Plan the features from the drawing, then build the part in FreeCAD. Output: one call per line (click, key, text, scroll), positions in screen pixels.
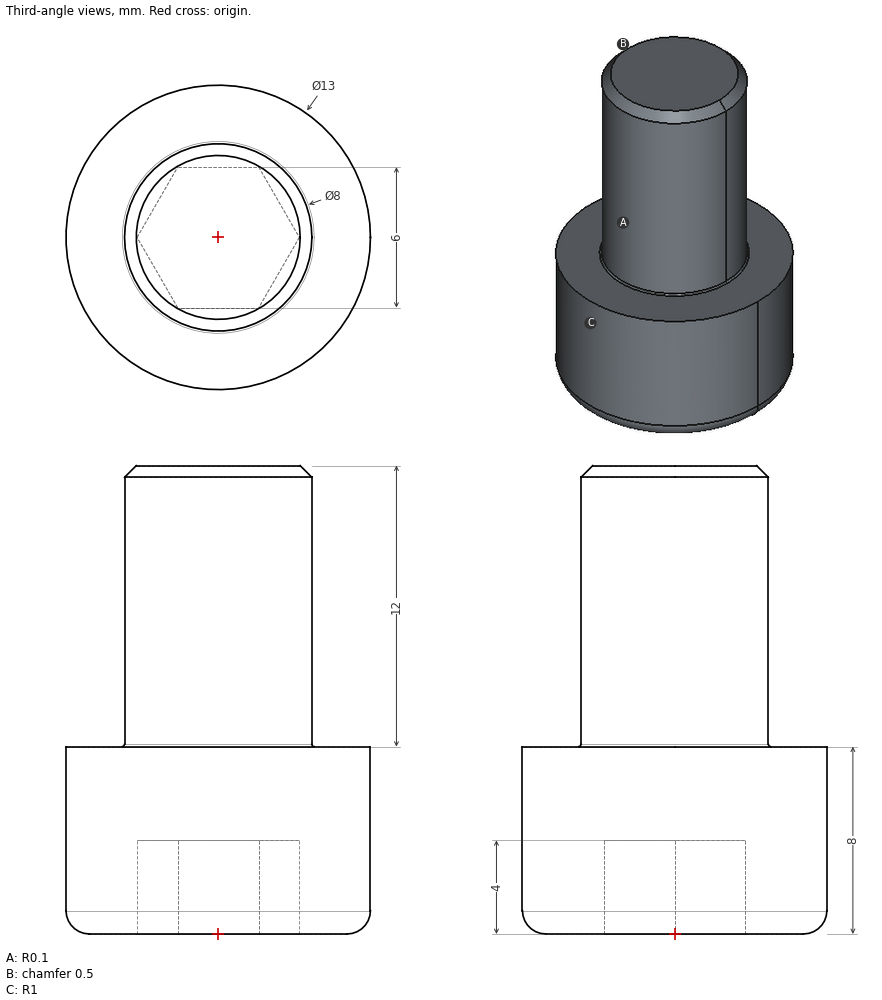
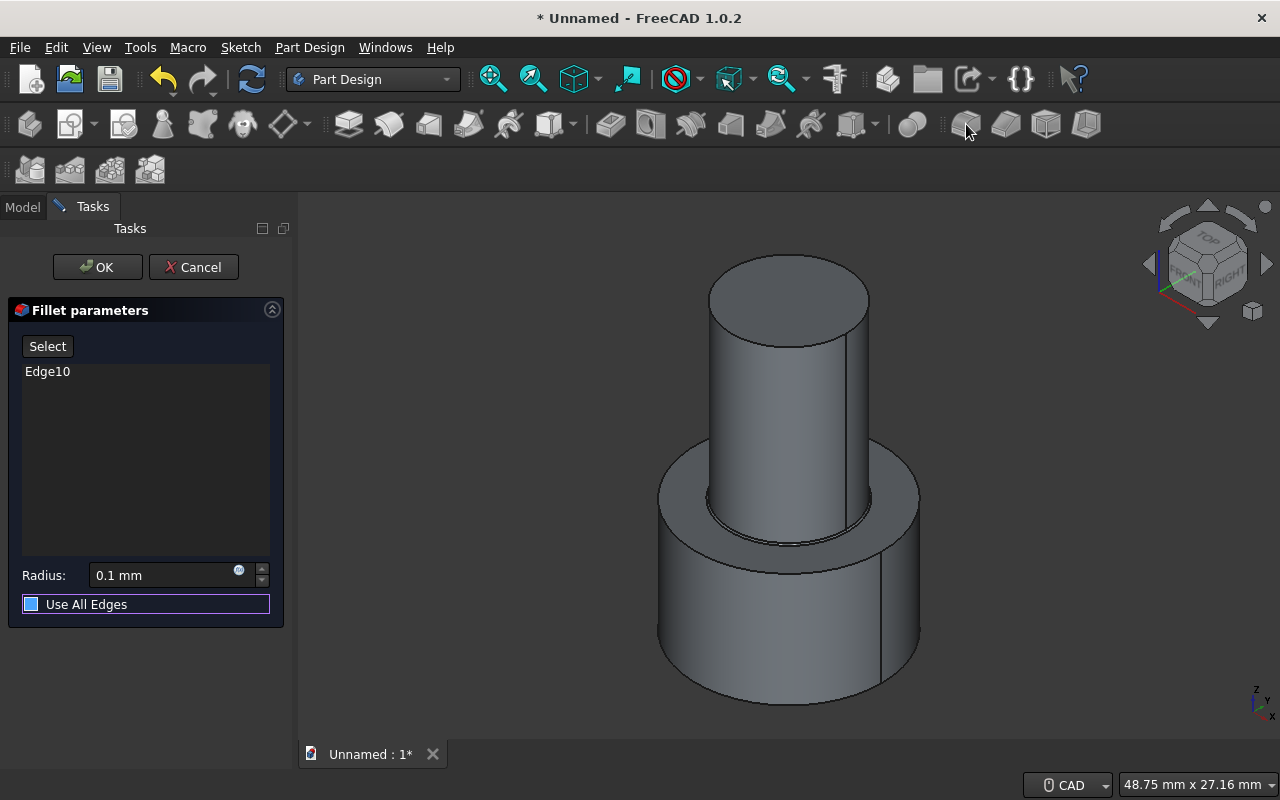
click(98, 267)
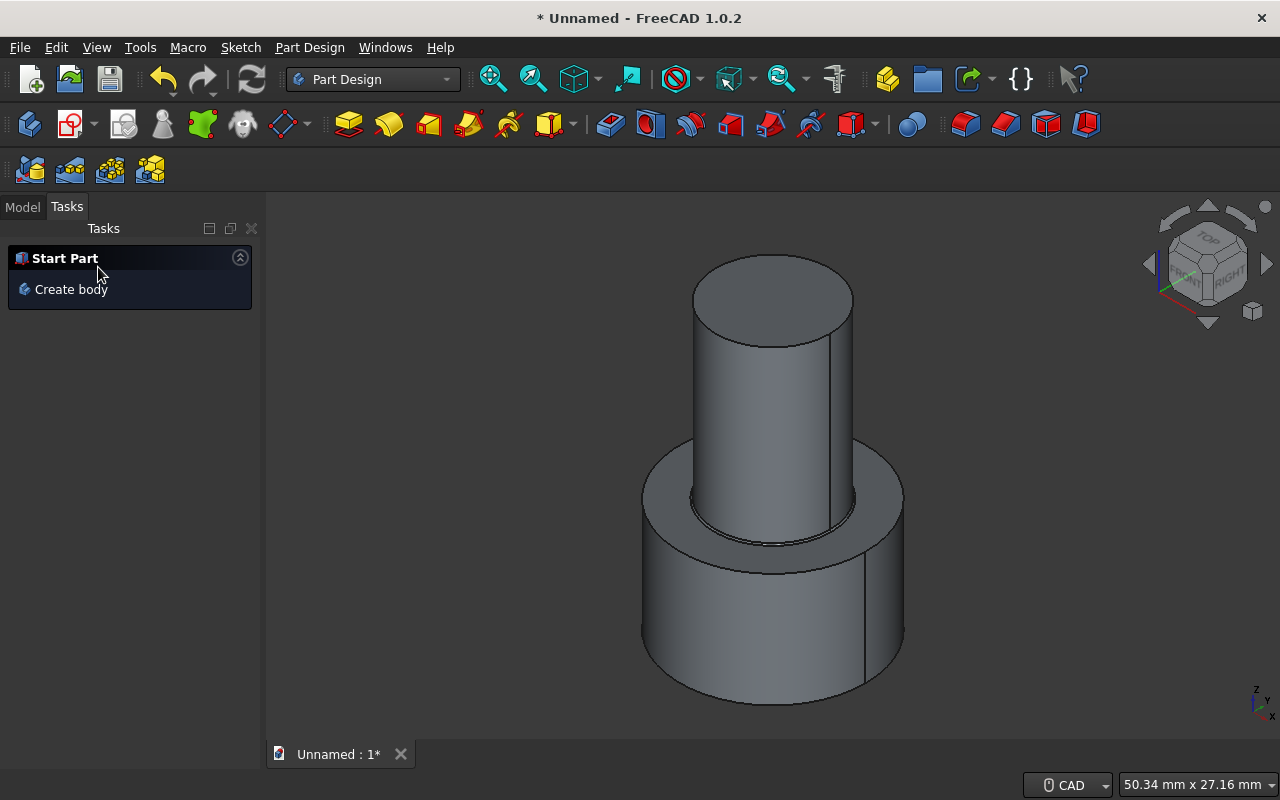
click(701, 321)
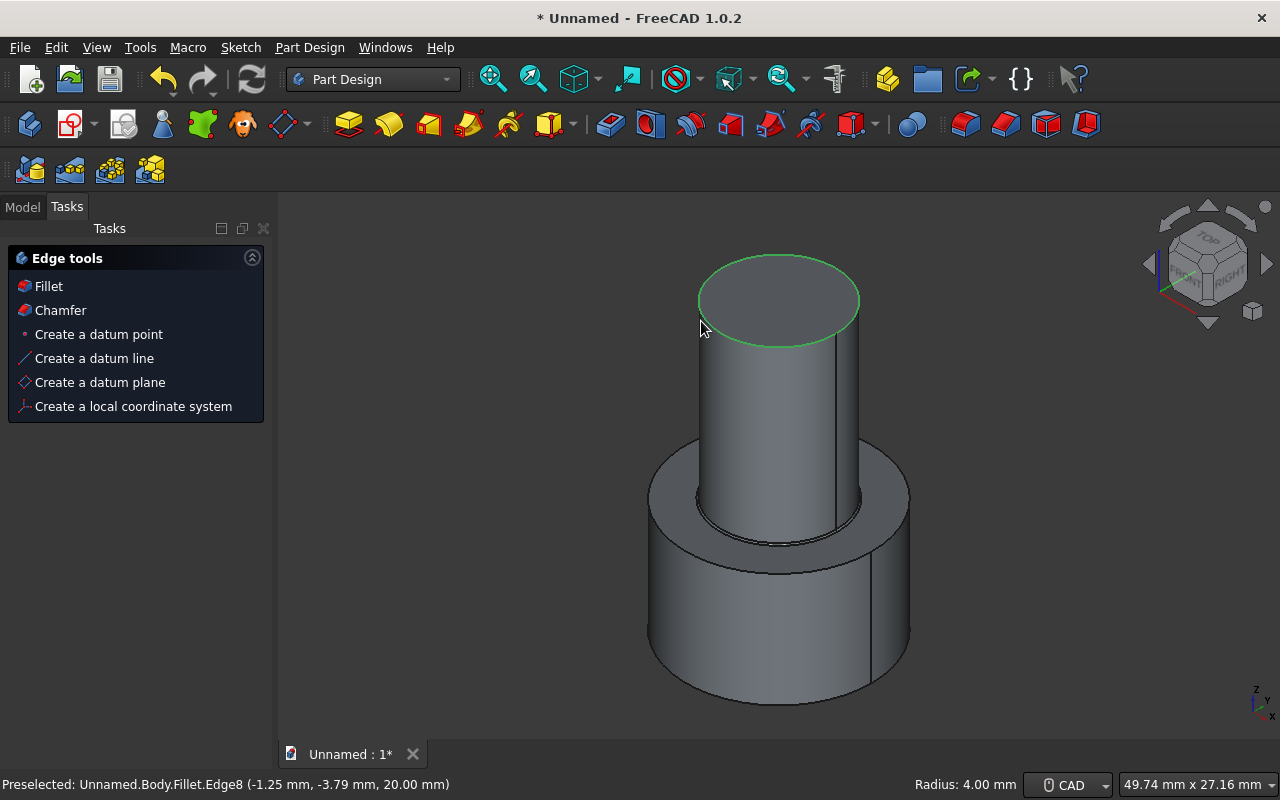
click(1006, 124)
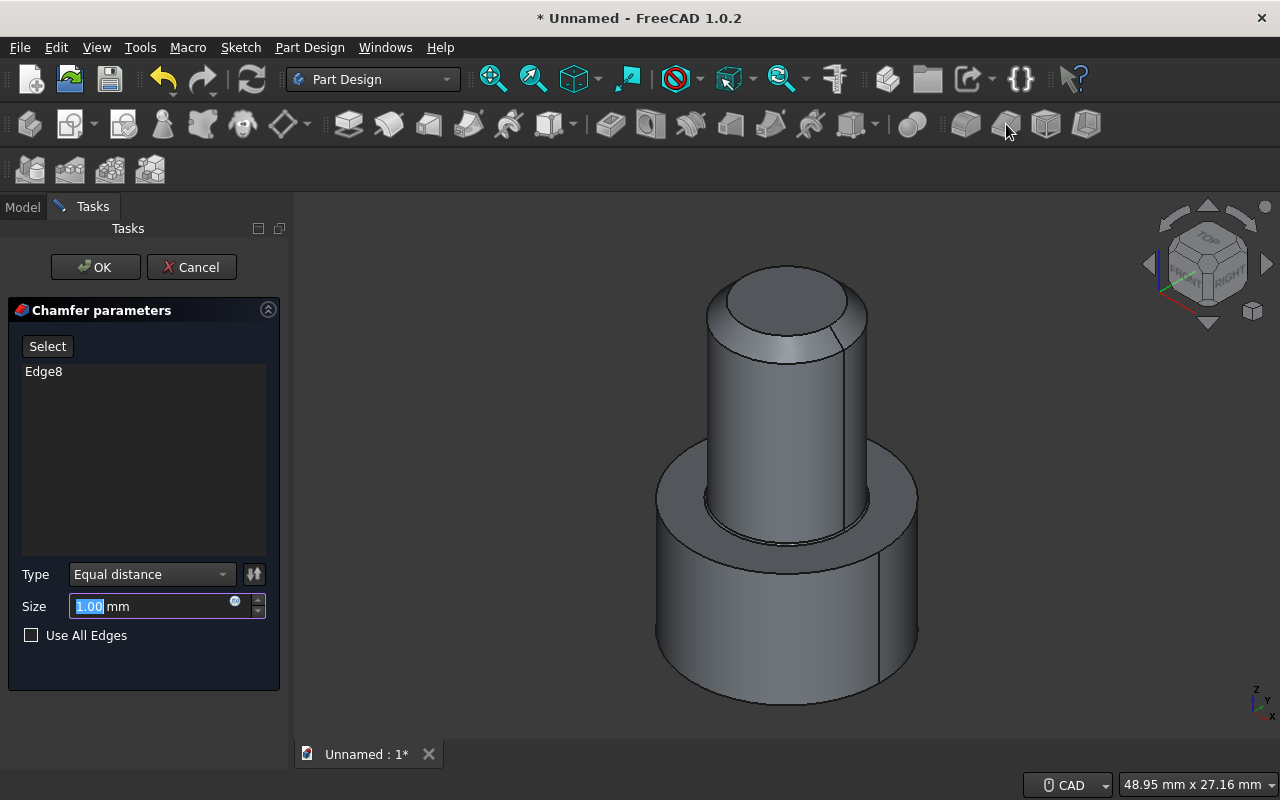
text(0.5)
key(Tab)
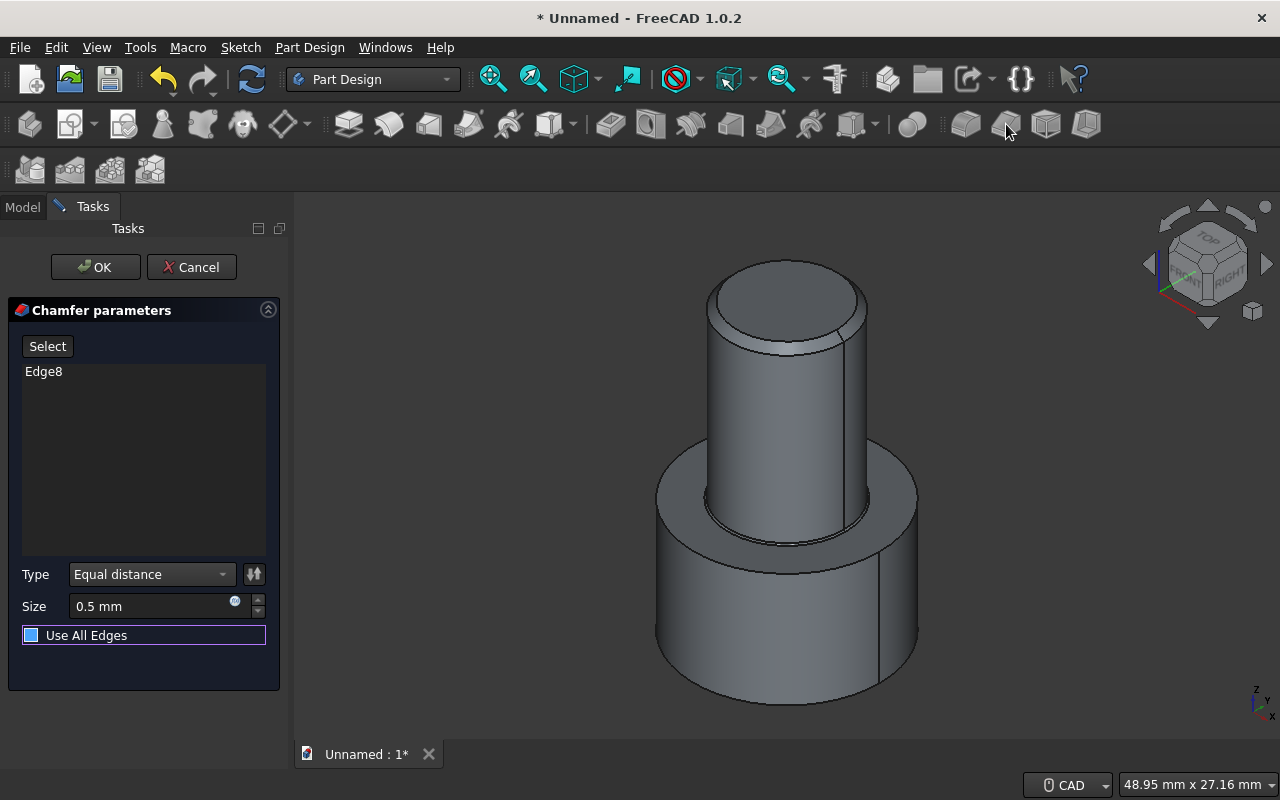
click(96, 267)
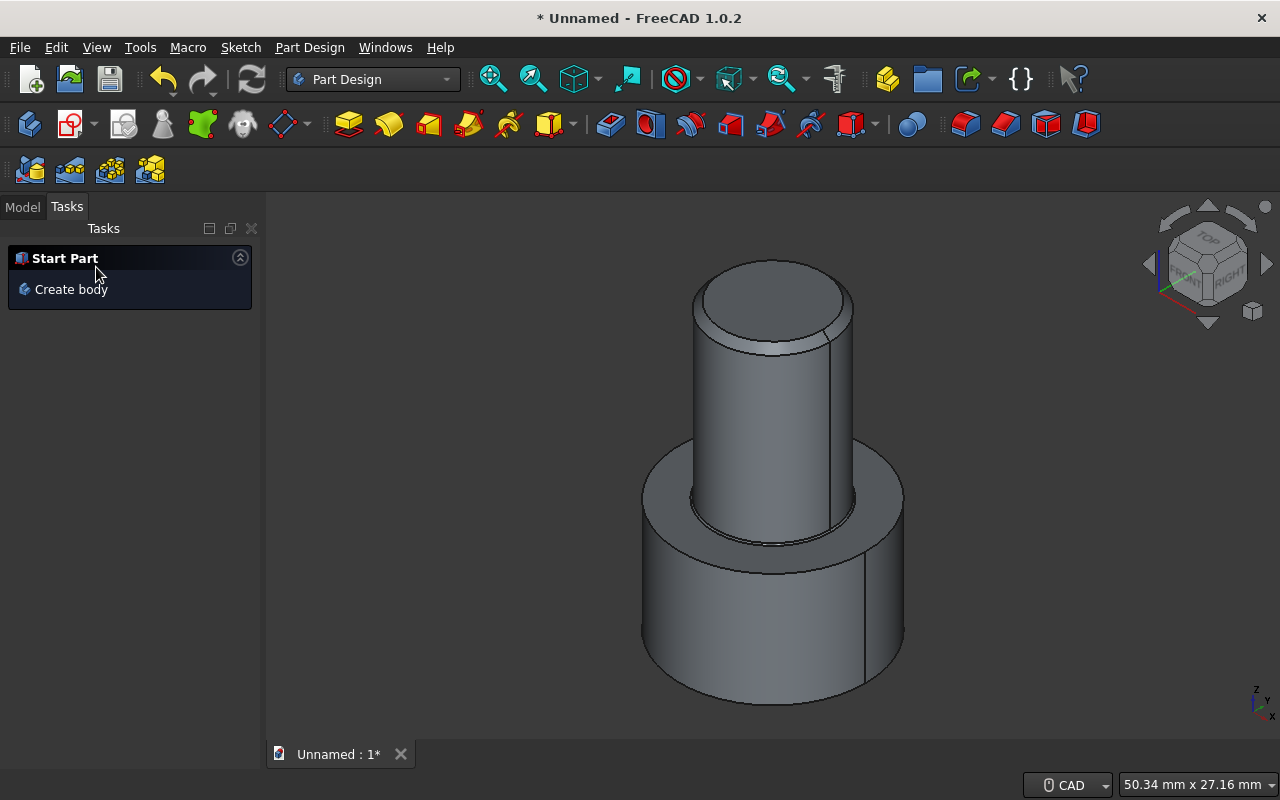
key(2)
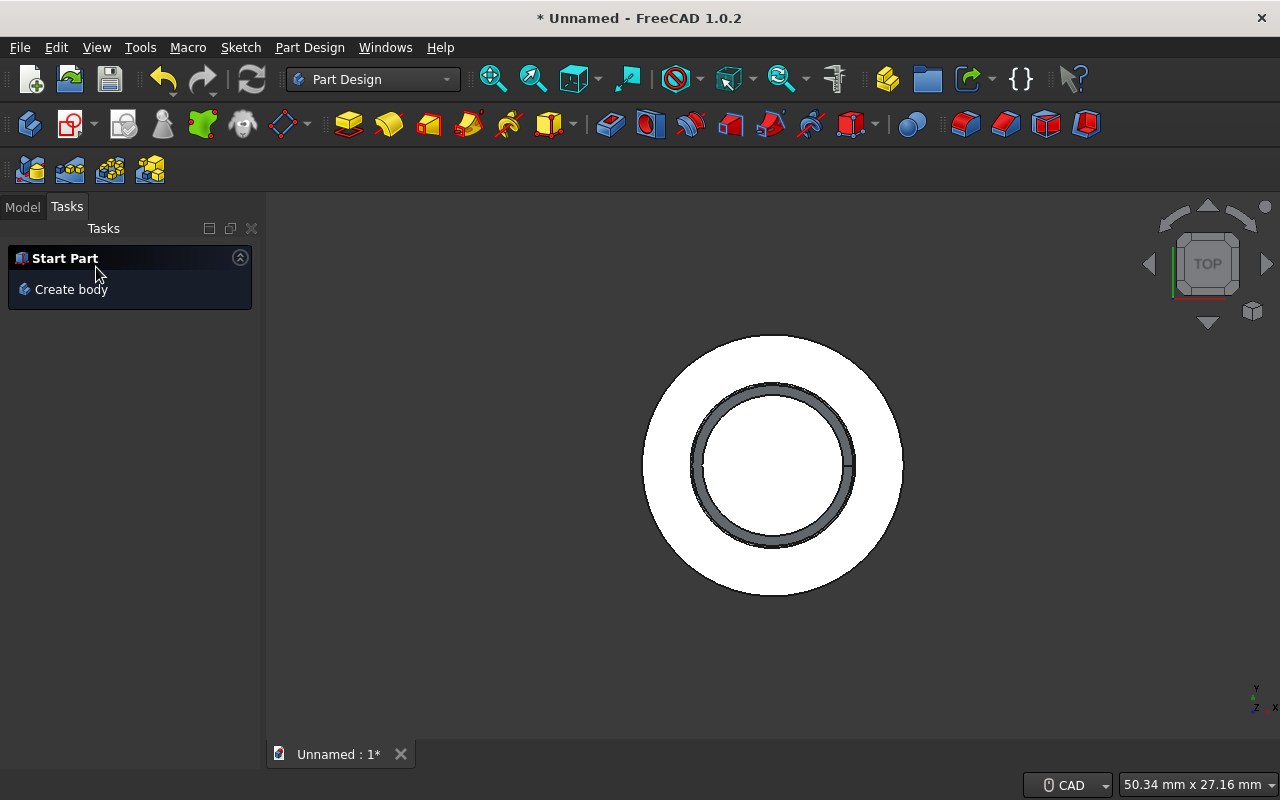
key(0)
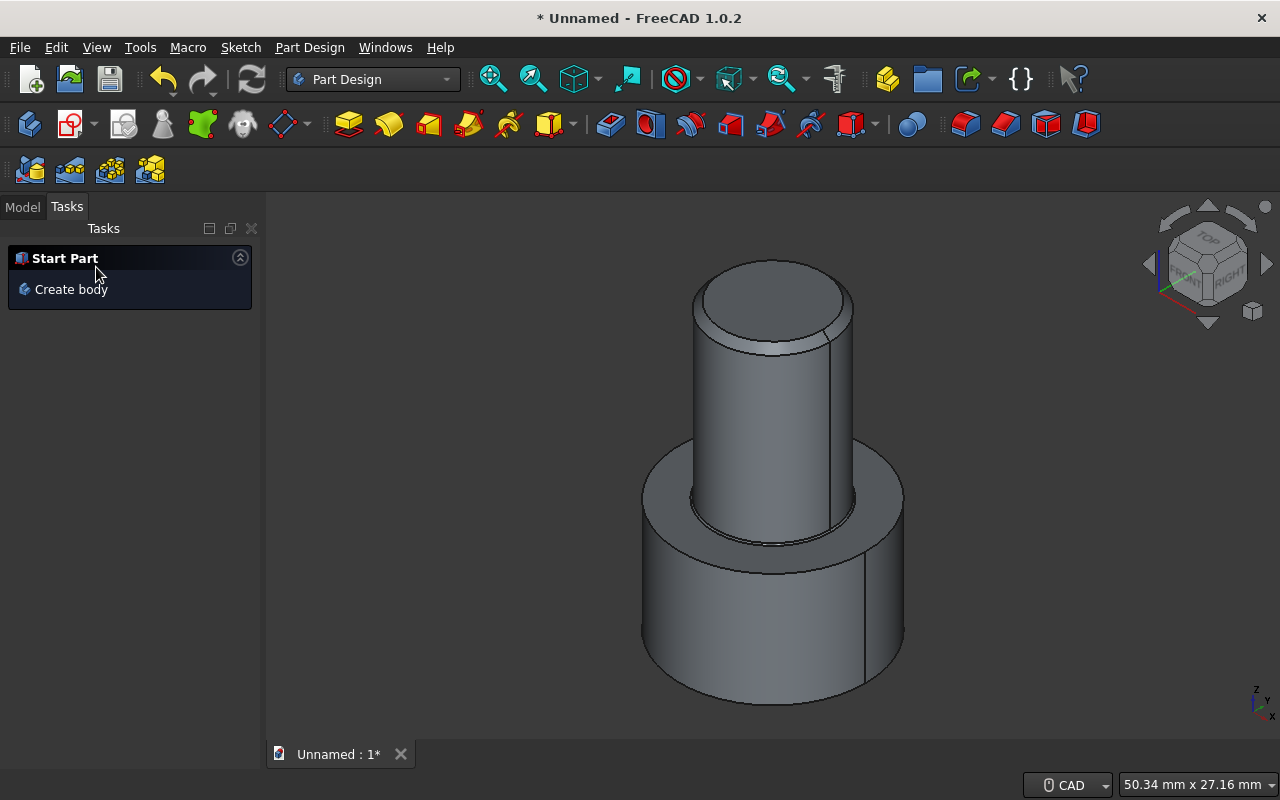
key(1)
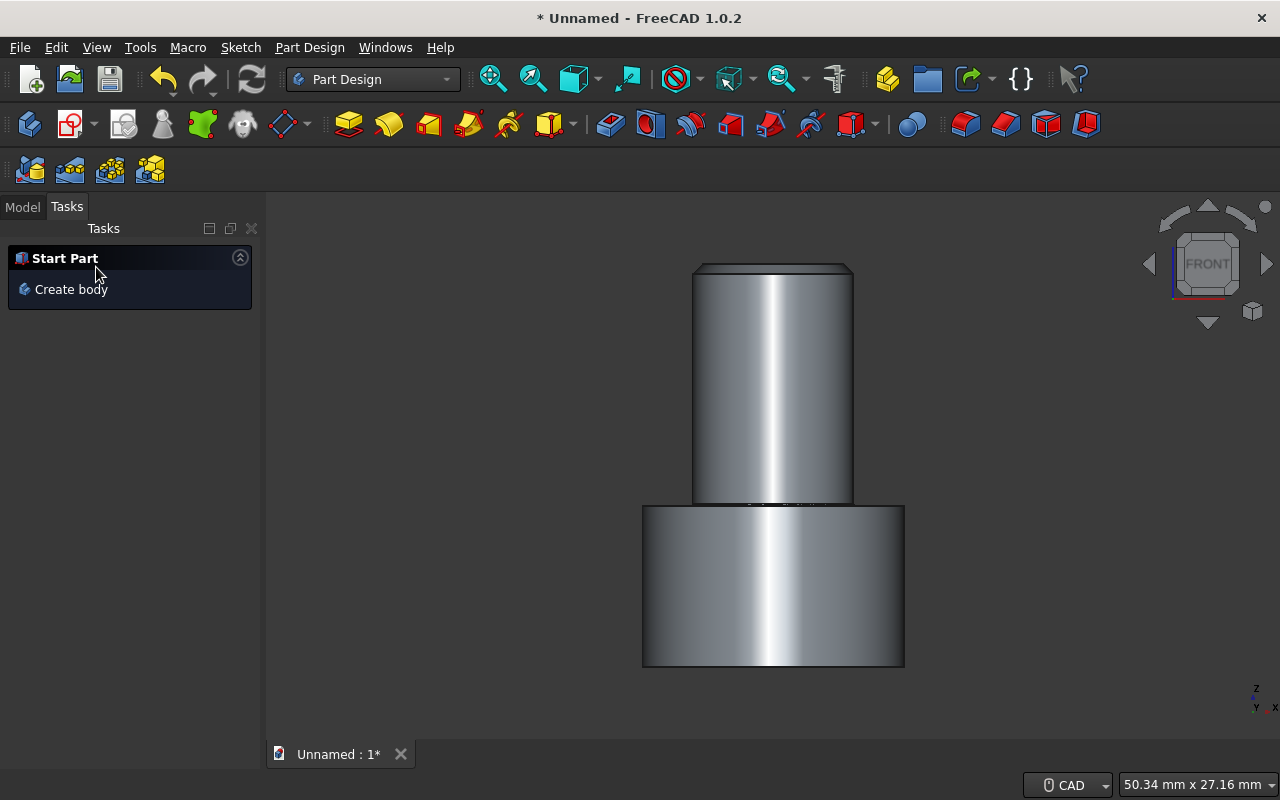
click(667, 666)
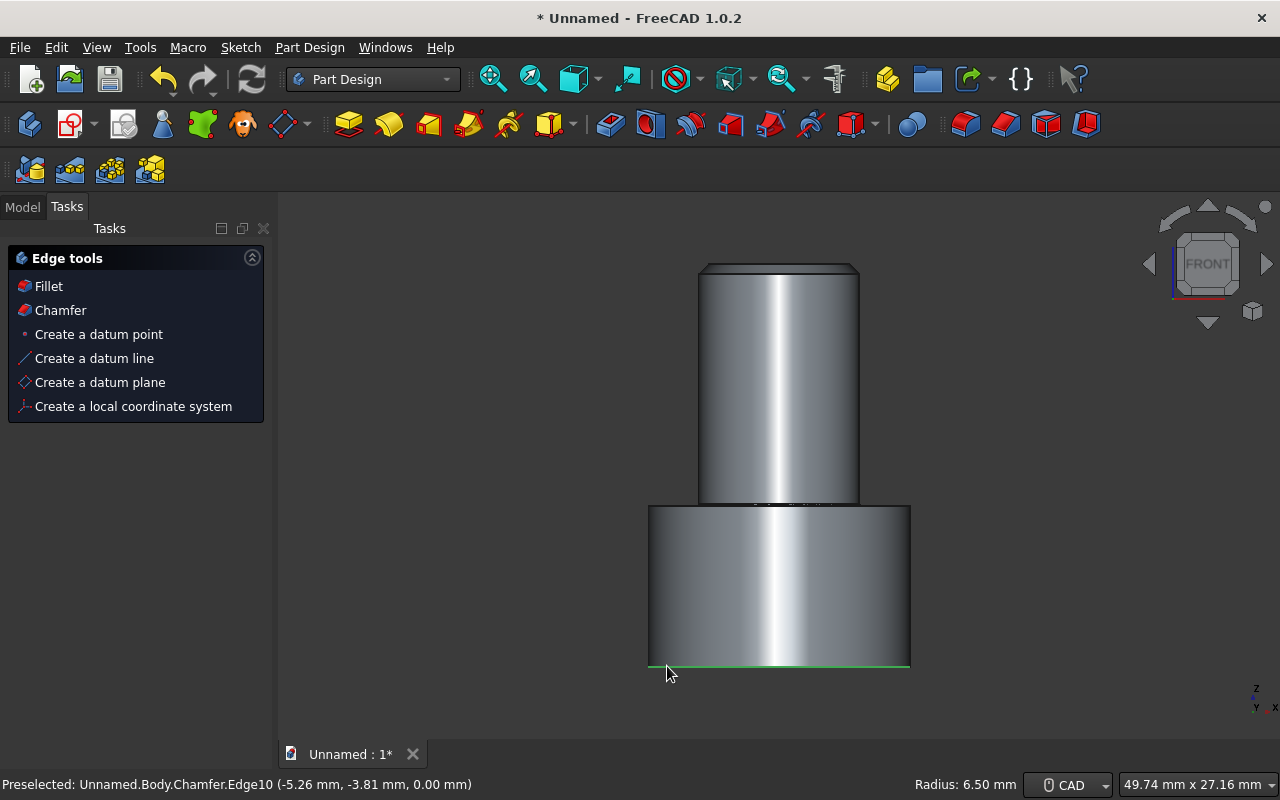
click(966, 124)